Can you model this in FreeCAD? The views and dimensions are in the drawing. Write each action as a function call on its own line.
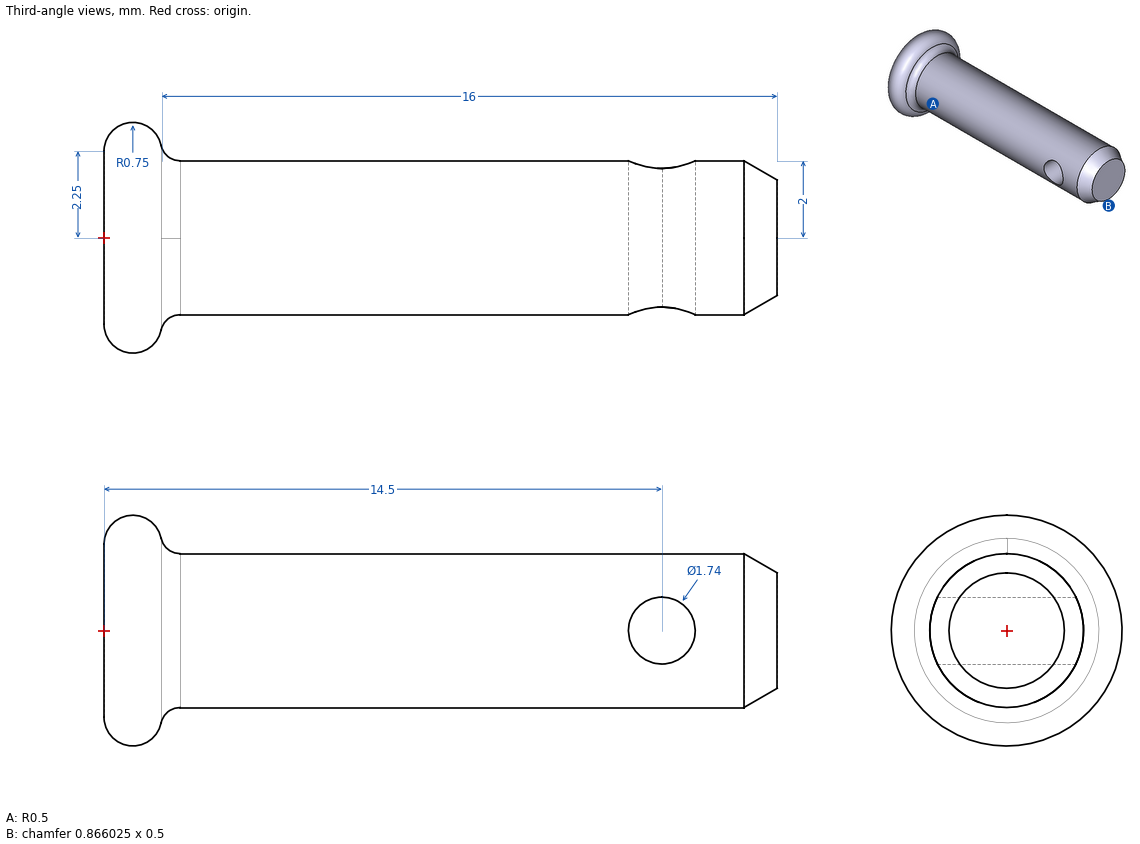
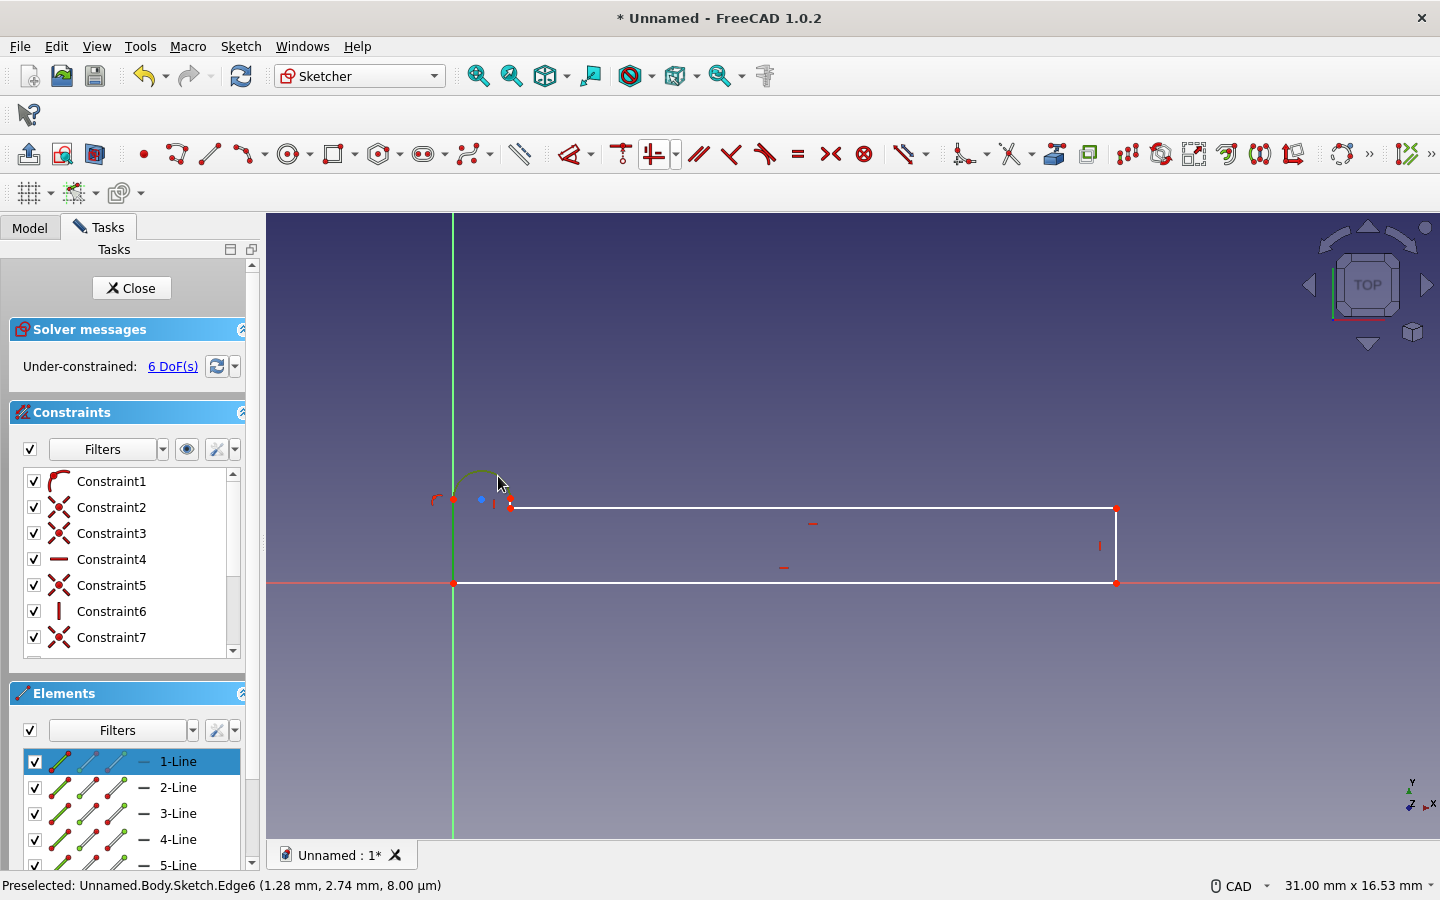
click(765, 154)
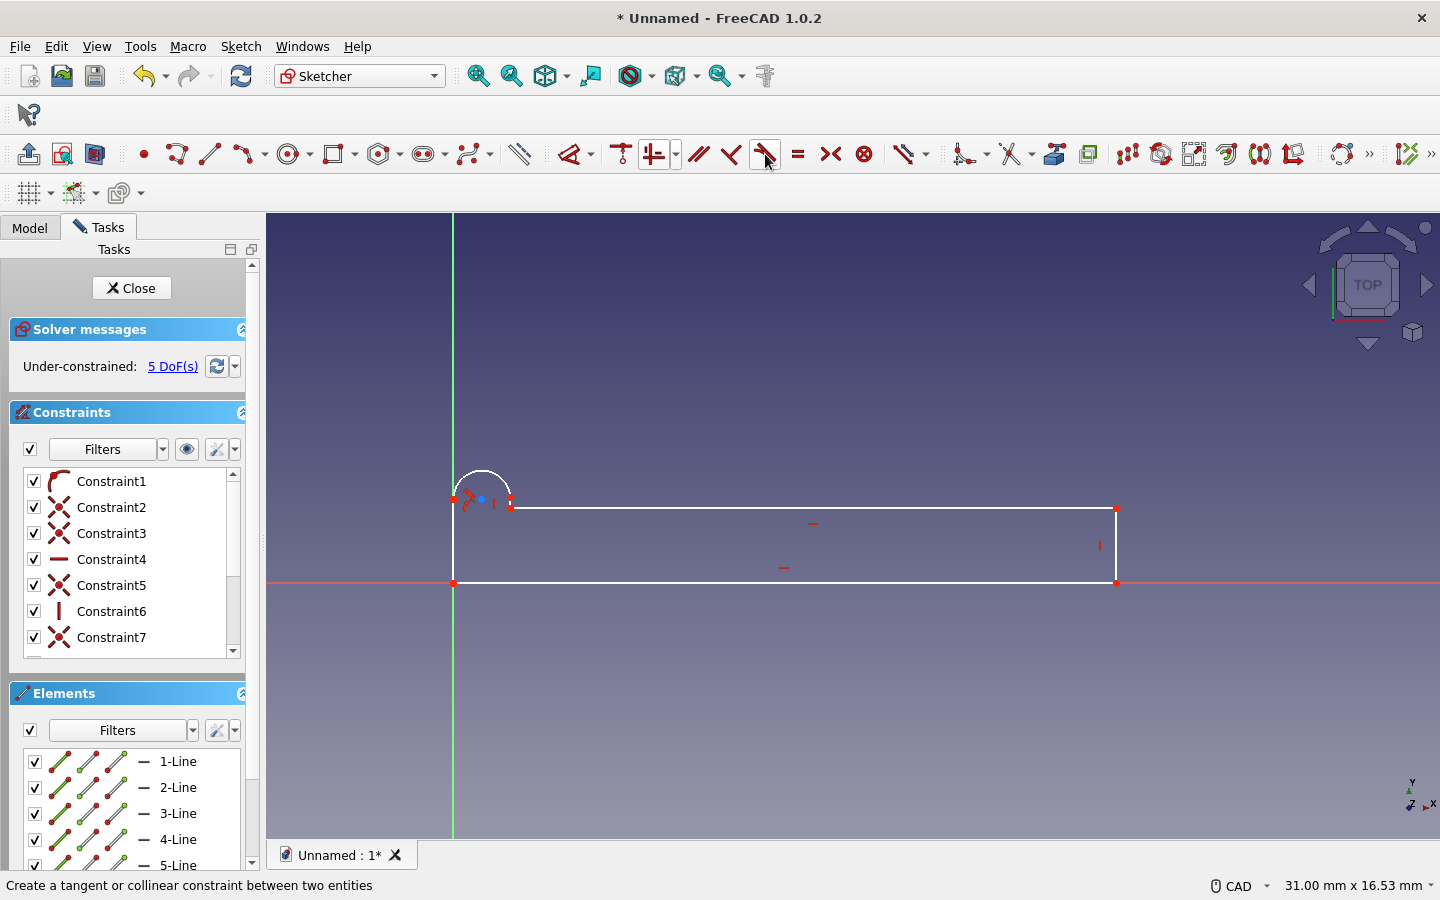
scroll(510, 503, up, 6)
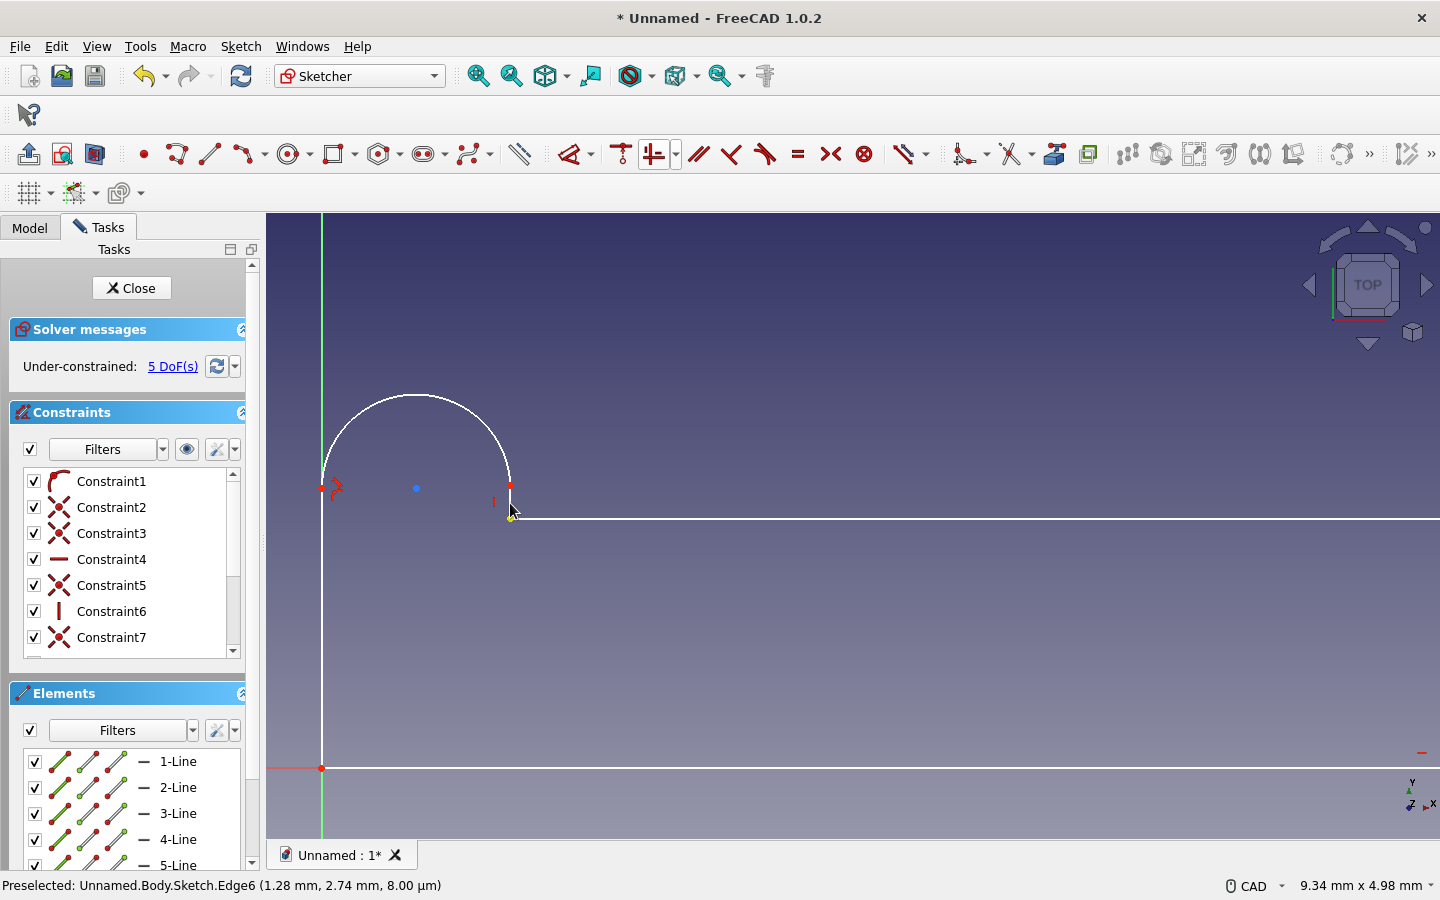
click(510, 502)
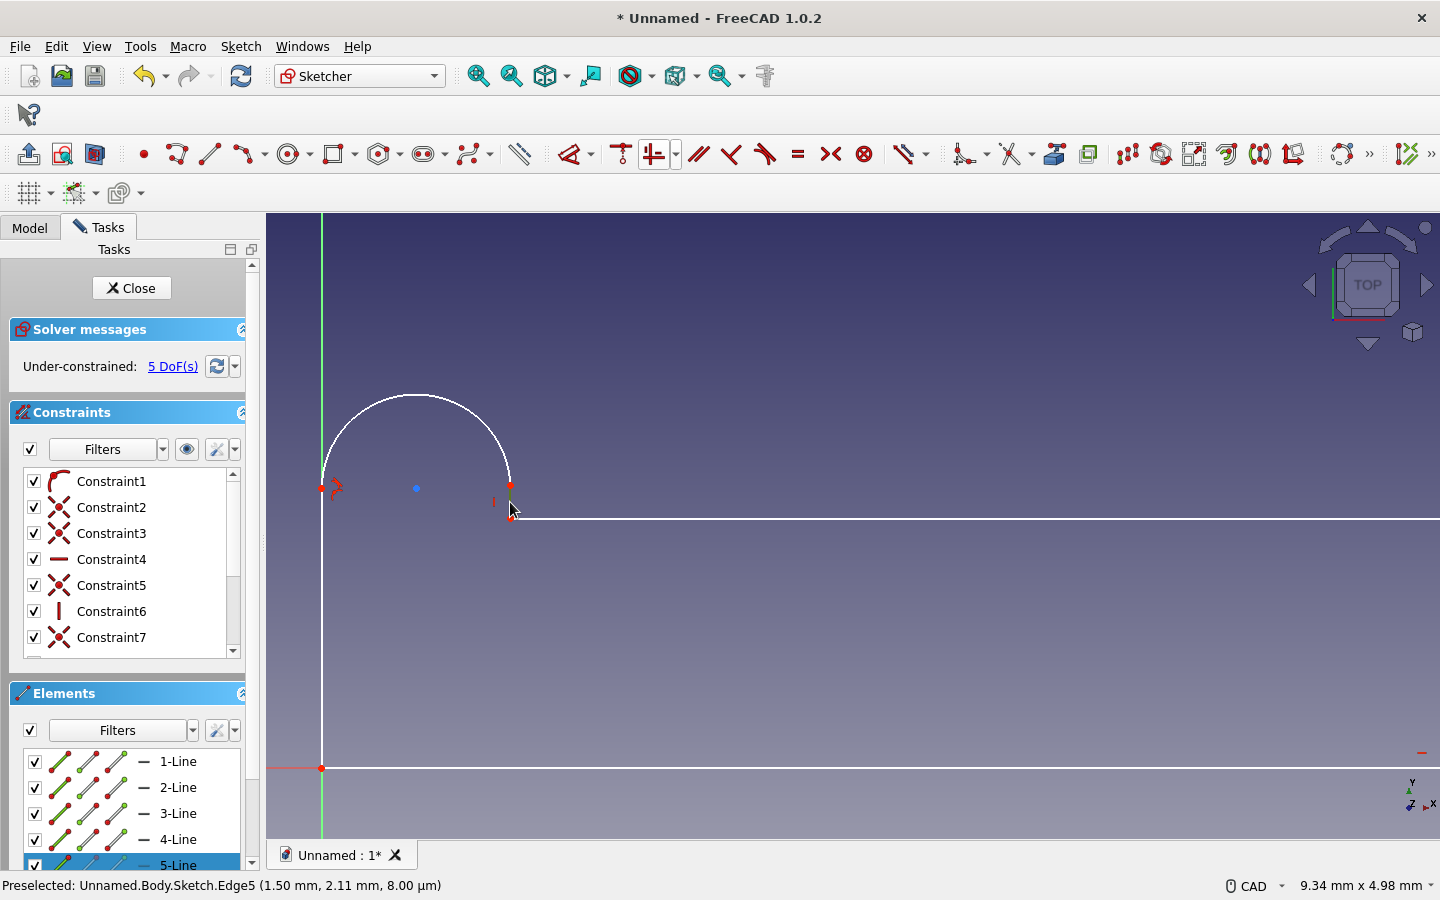
click(469, 411)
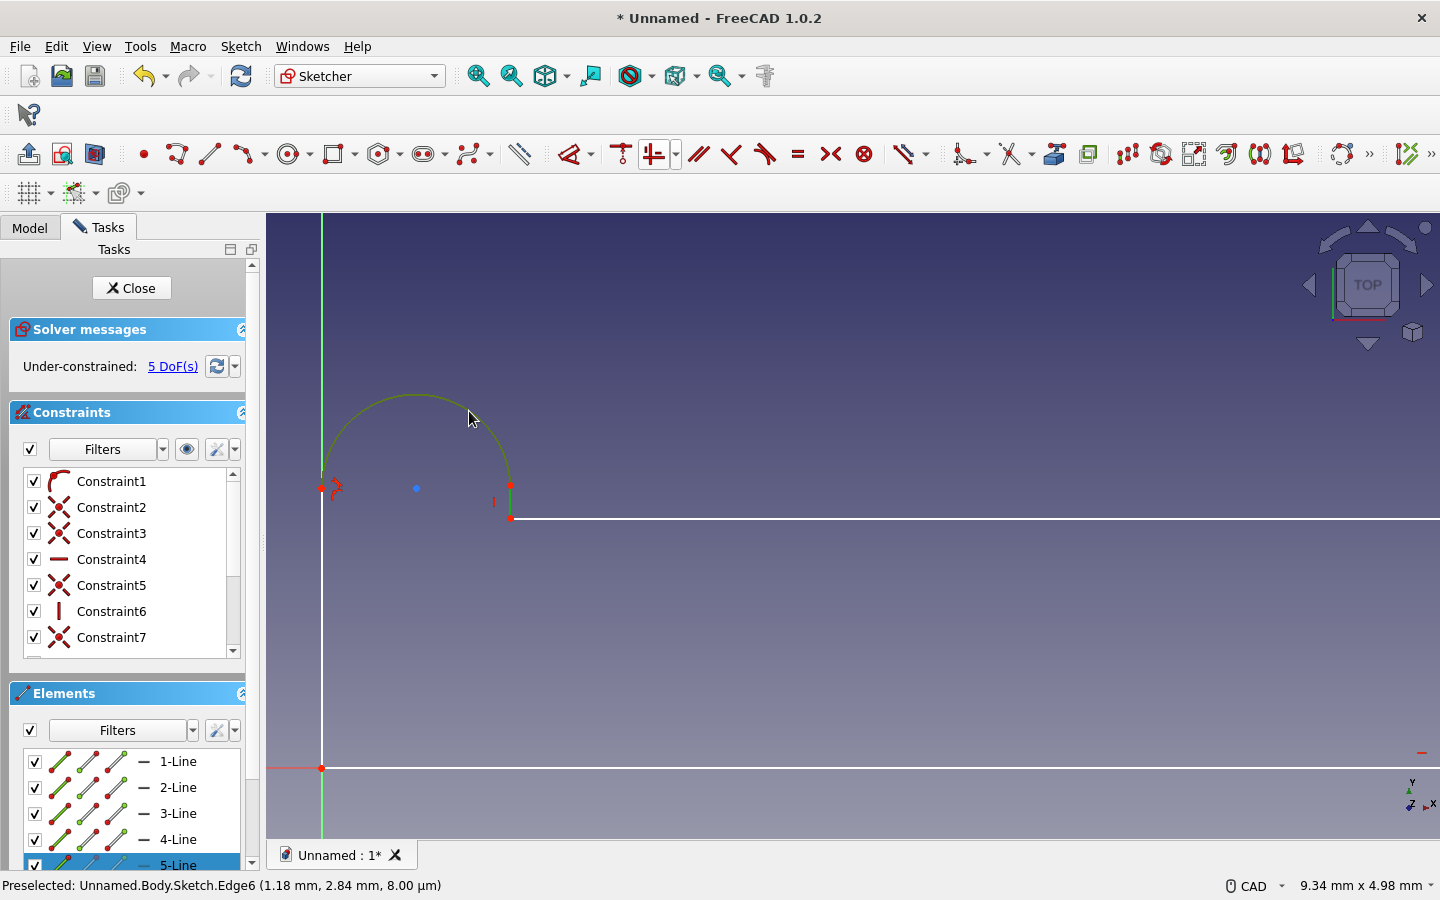
click(765, 154)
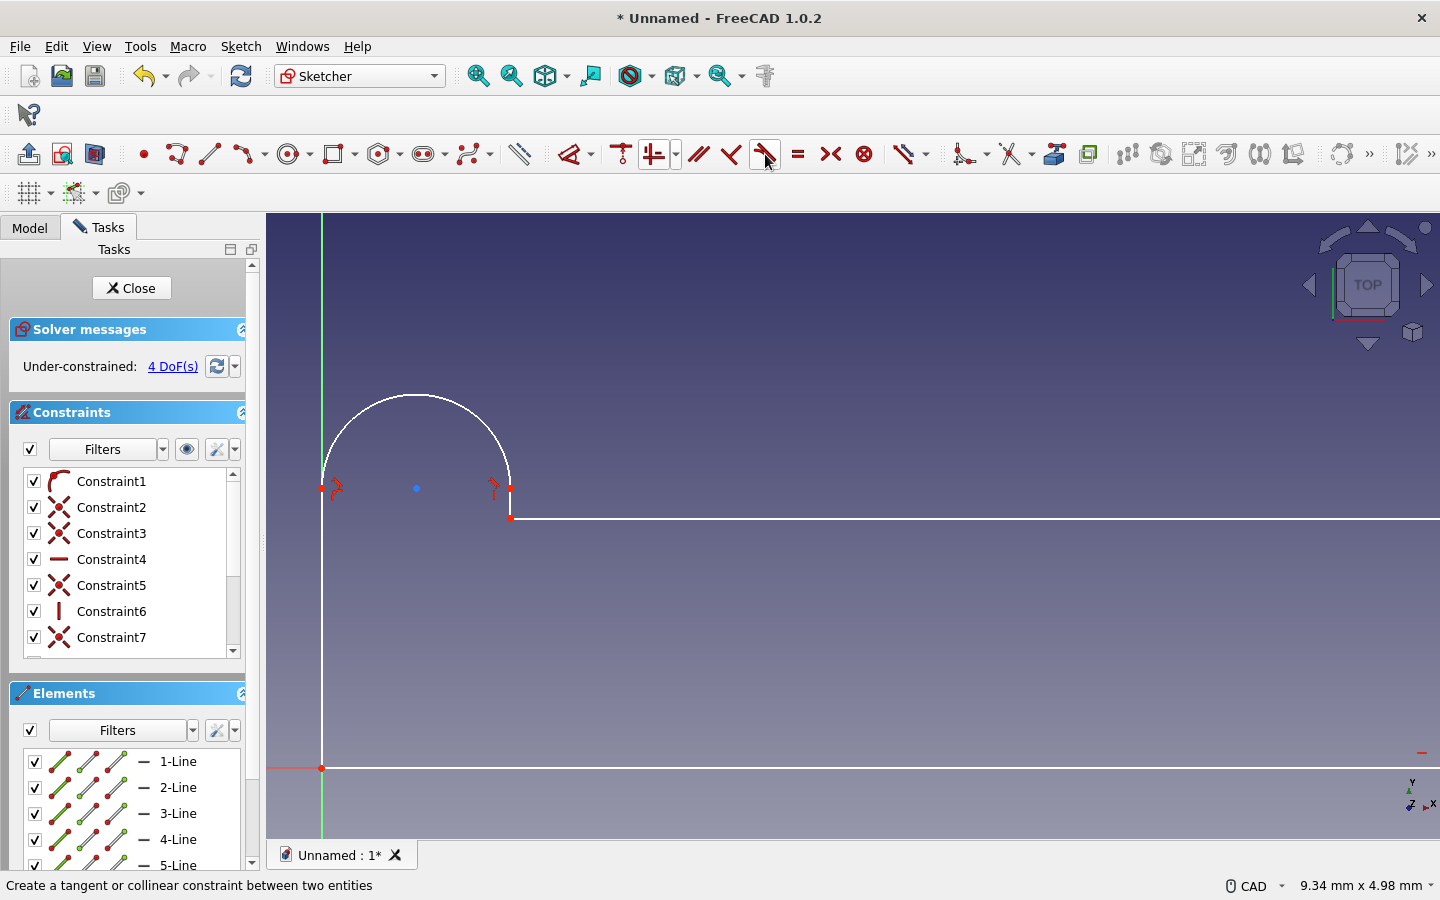
click(568, 154)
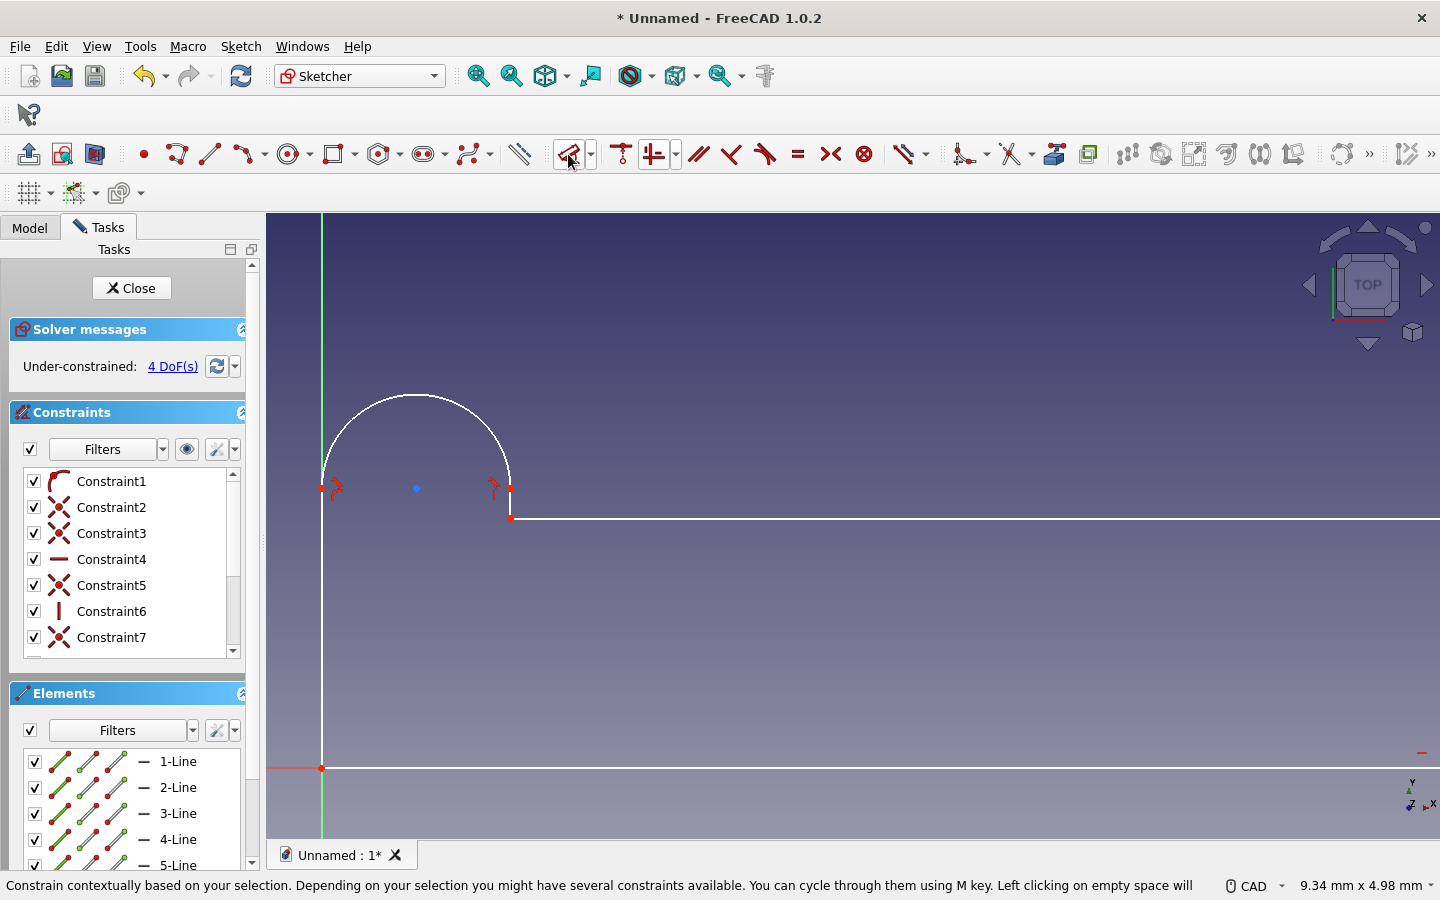
click(472, 413)
click(491, 387)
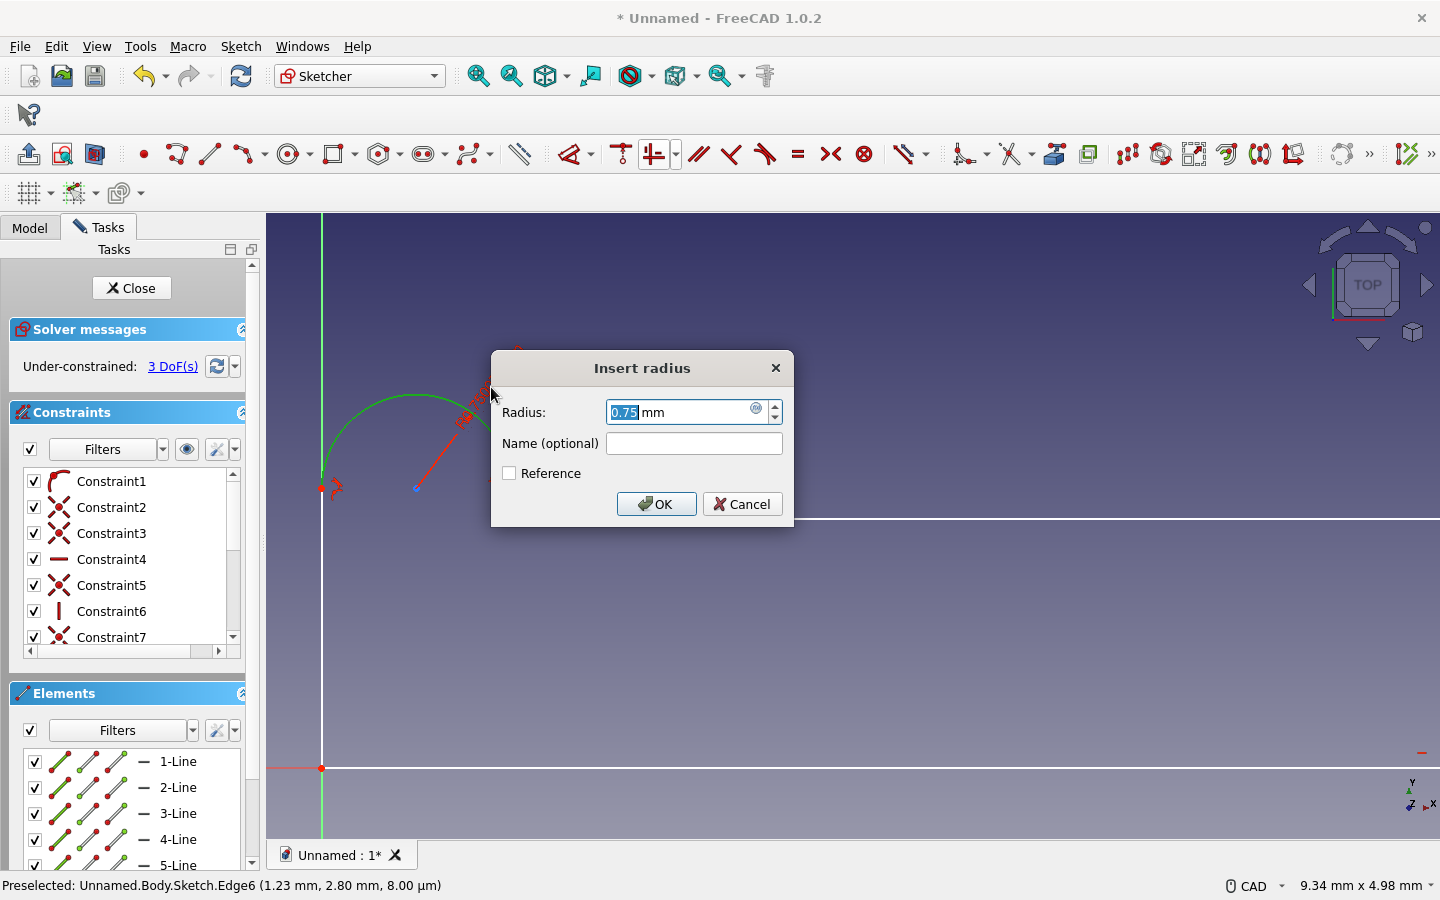
text(0.75)
key(Return)